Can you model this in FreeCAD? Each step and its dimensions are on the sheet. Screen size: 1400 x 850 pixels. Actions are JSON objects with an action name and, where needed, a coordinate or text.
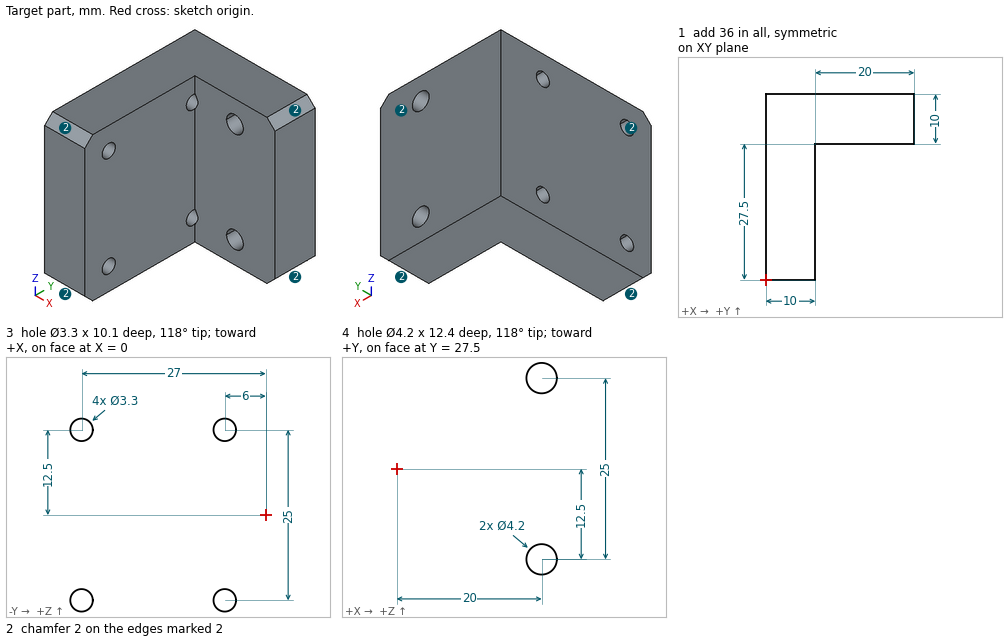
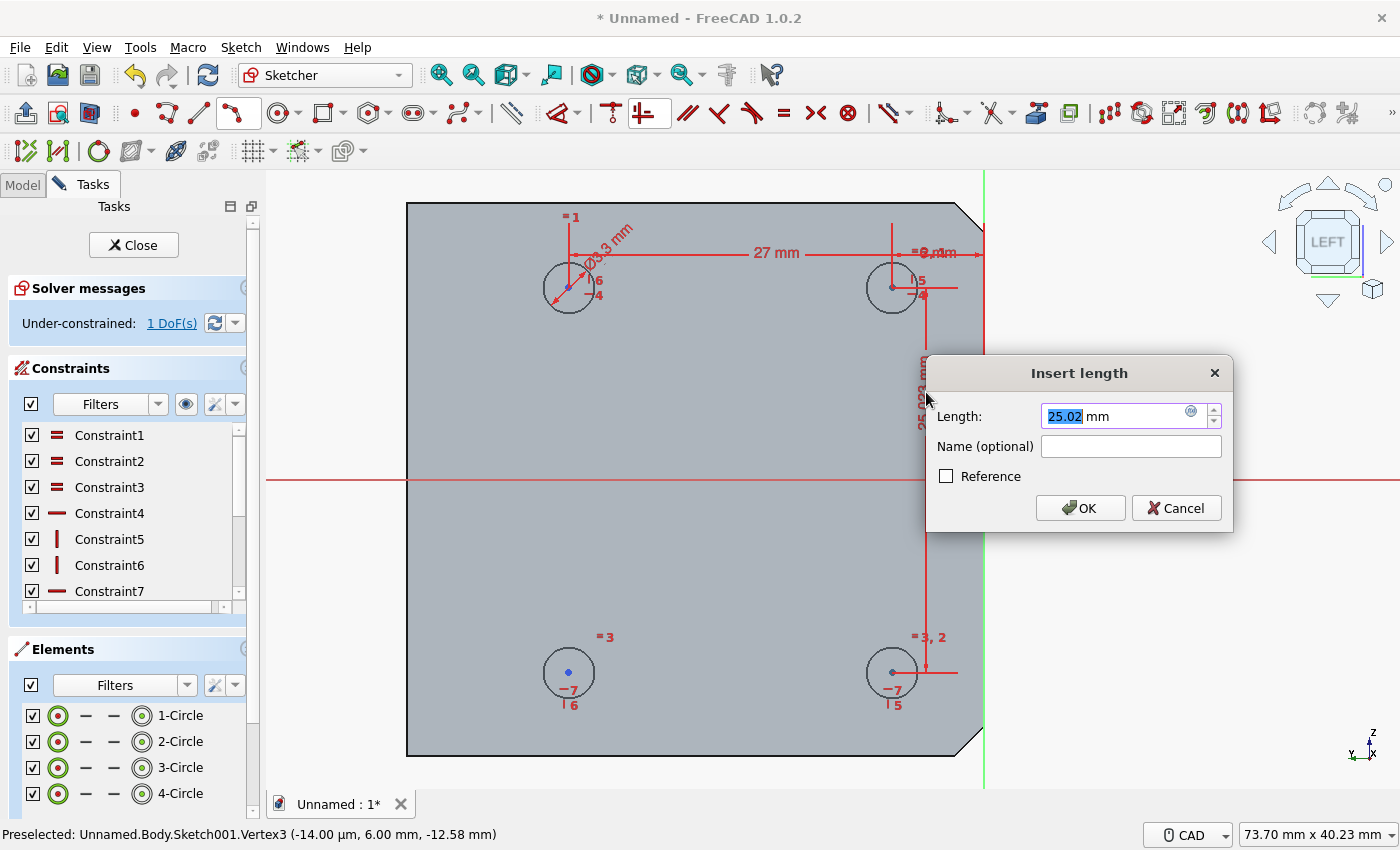
{"action": "type", "text": "25"}
{"action": "key", "text": "Return"}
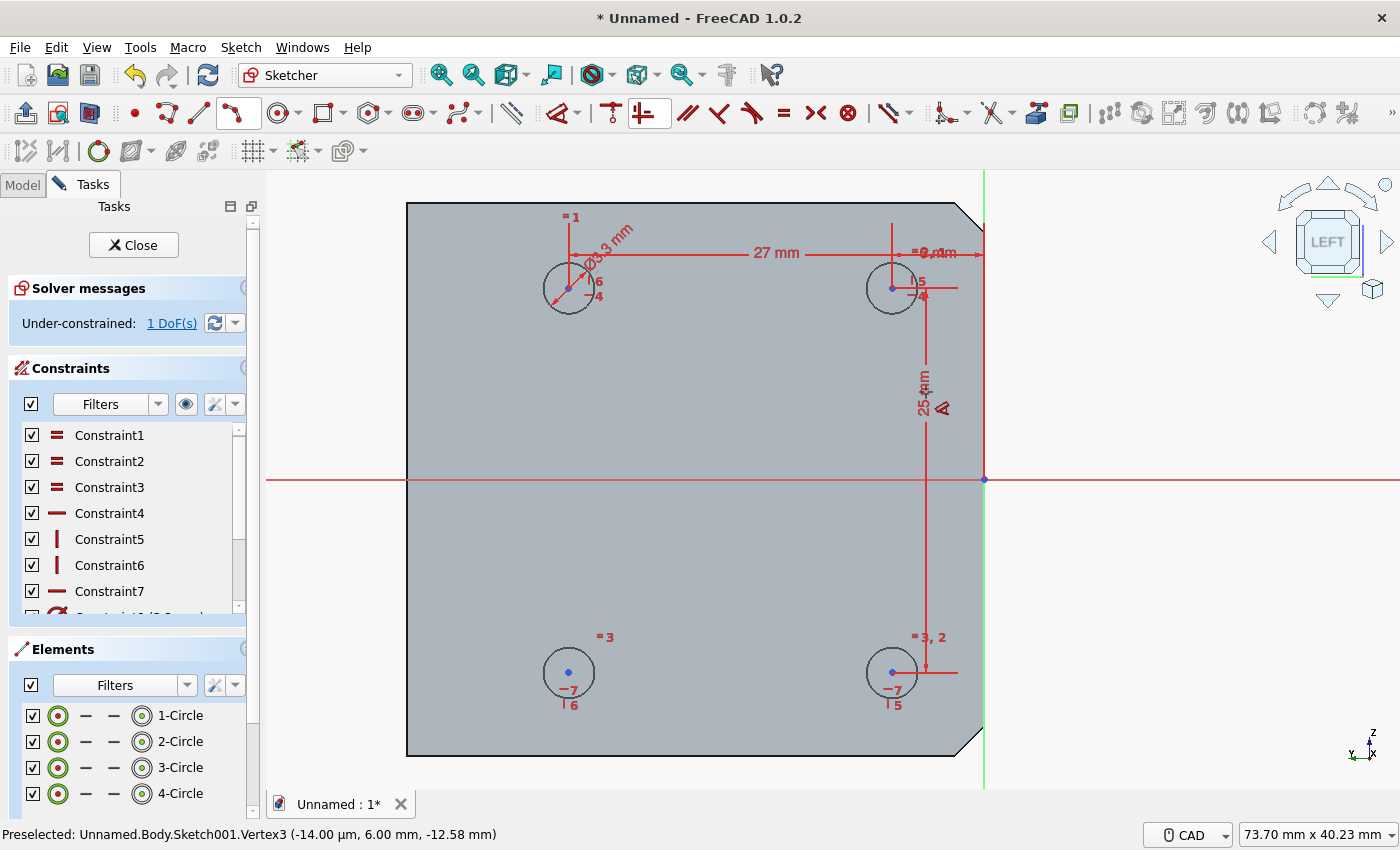
{"action": "left_click", "coordinate": [569, 288]}
{"action": "left_click", "coordinate": [1018, 384]}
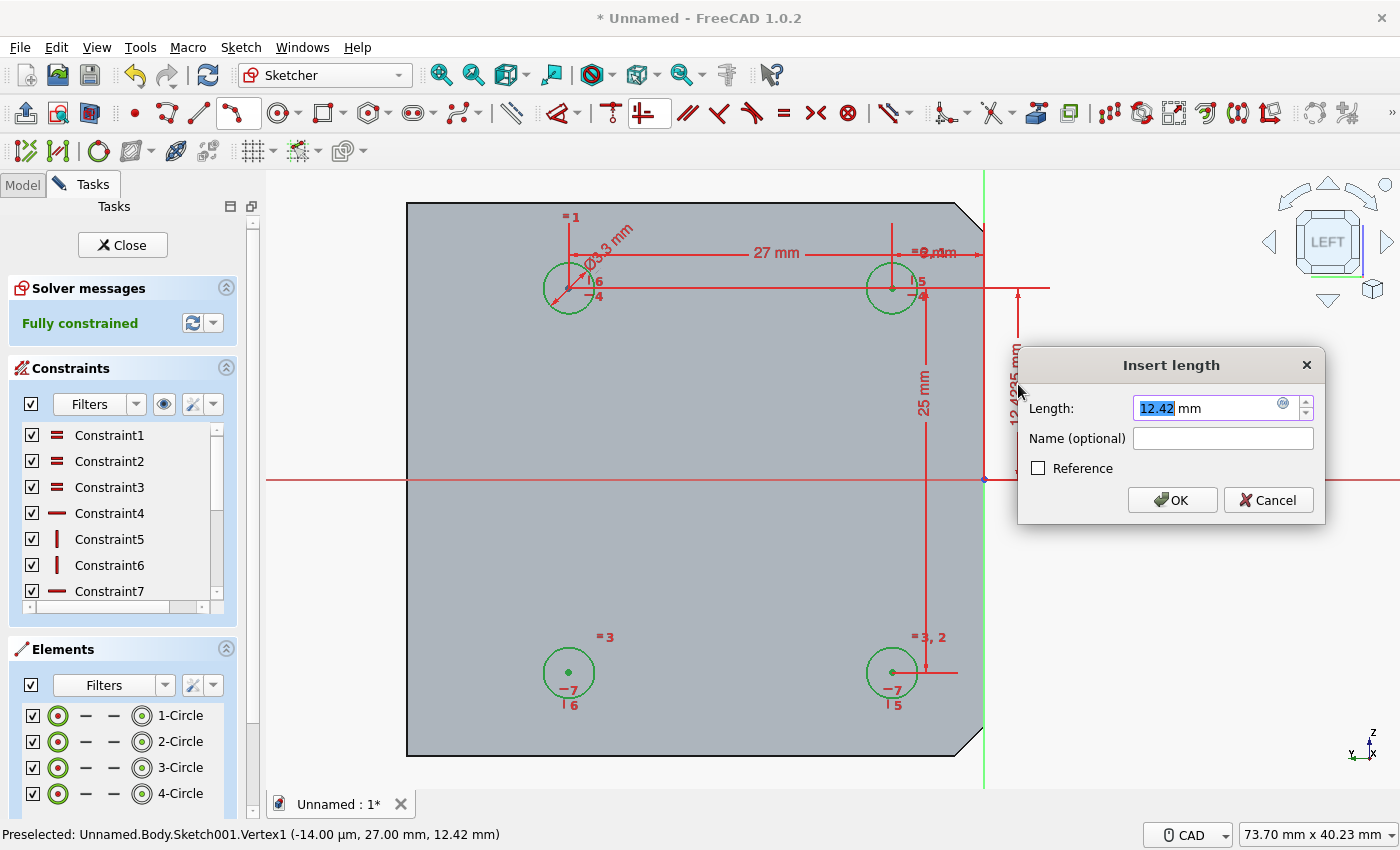
{"action": "type", "text": "12.5"}
{"action": "key", "text": "Return"}
{"action": "key", "text": "Escape"}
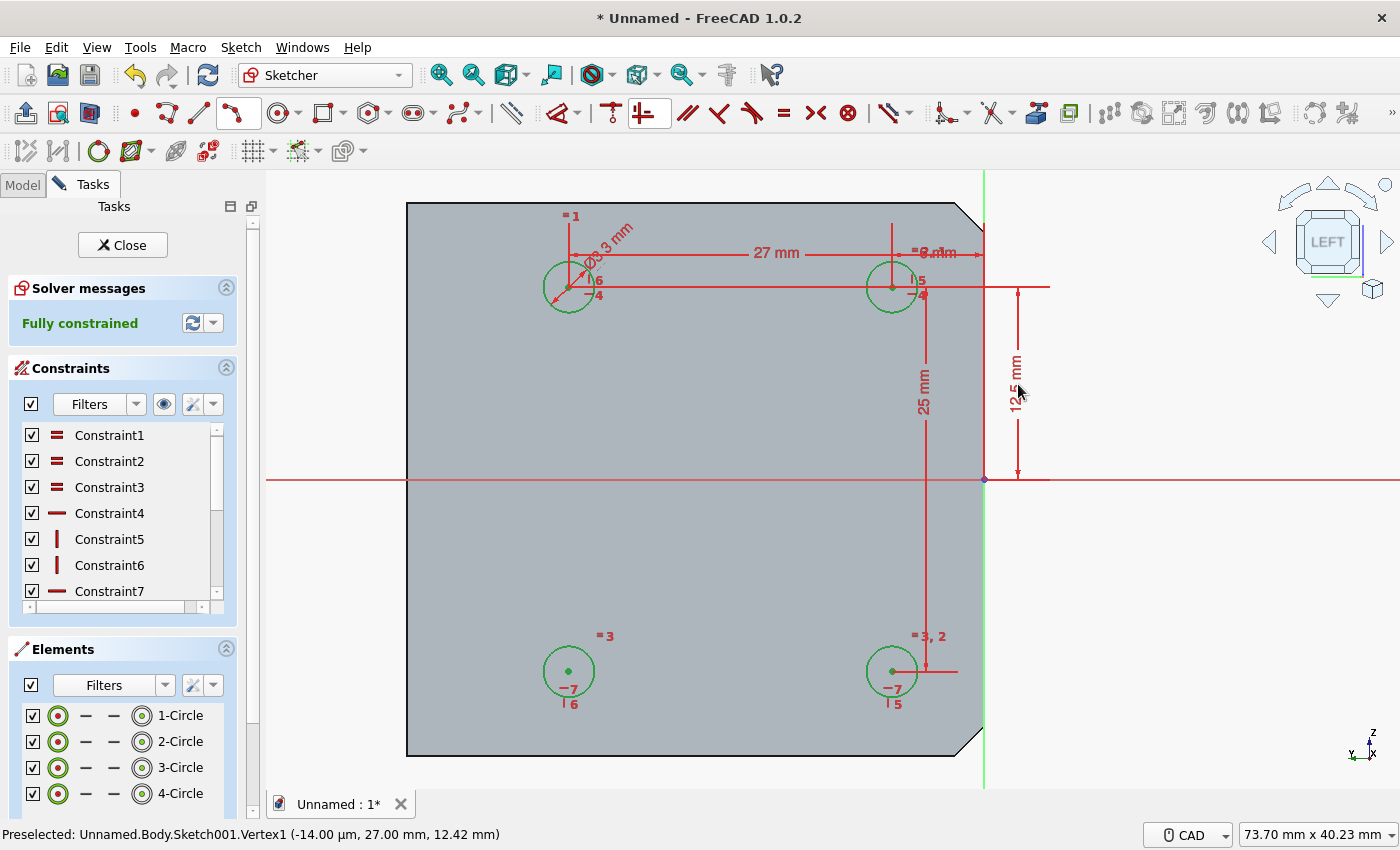
{"action": "left_click", "coordinate": [123, 245]}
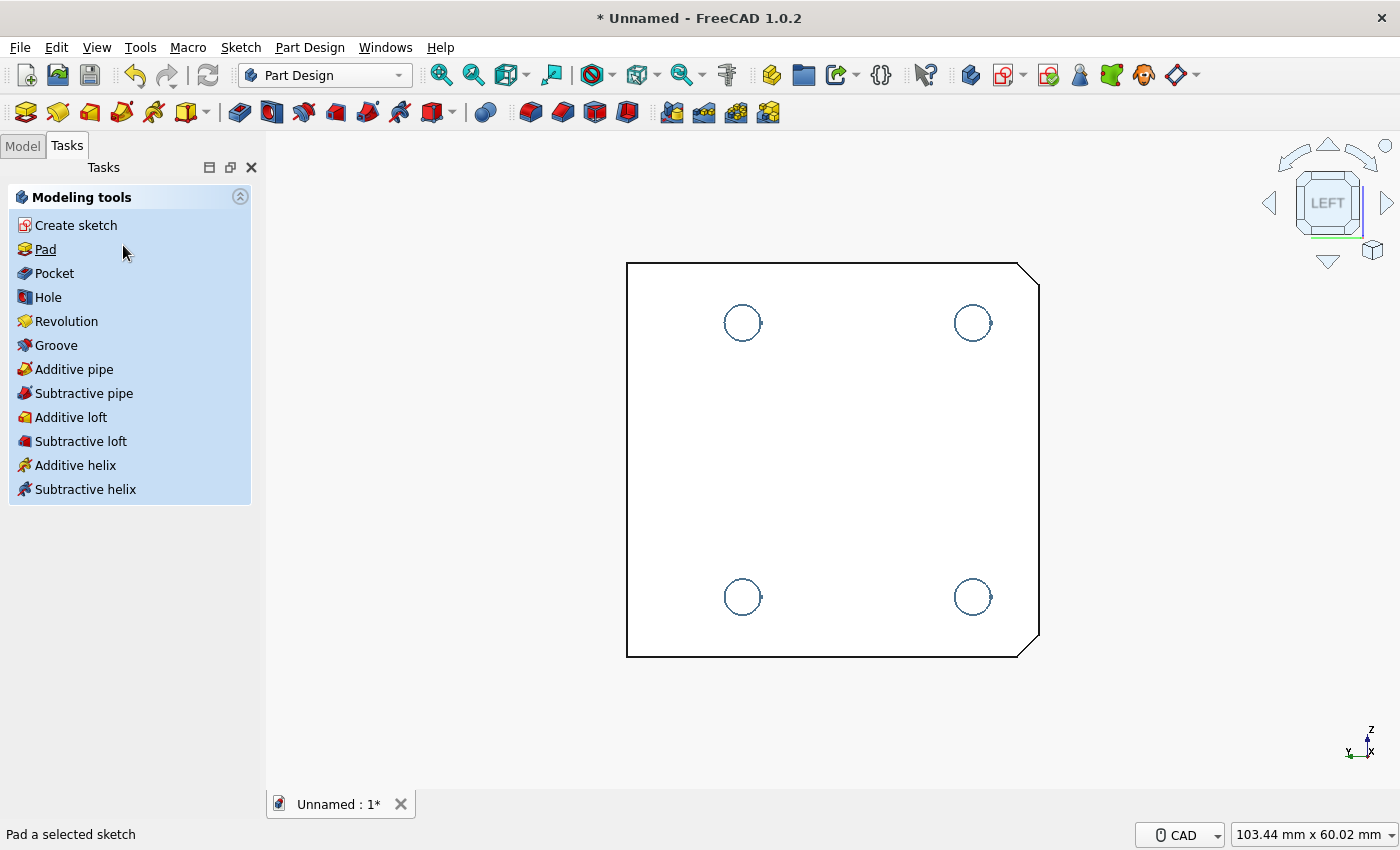
{"action": "left_click", "coordinate": [272, 112]}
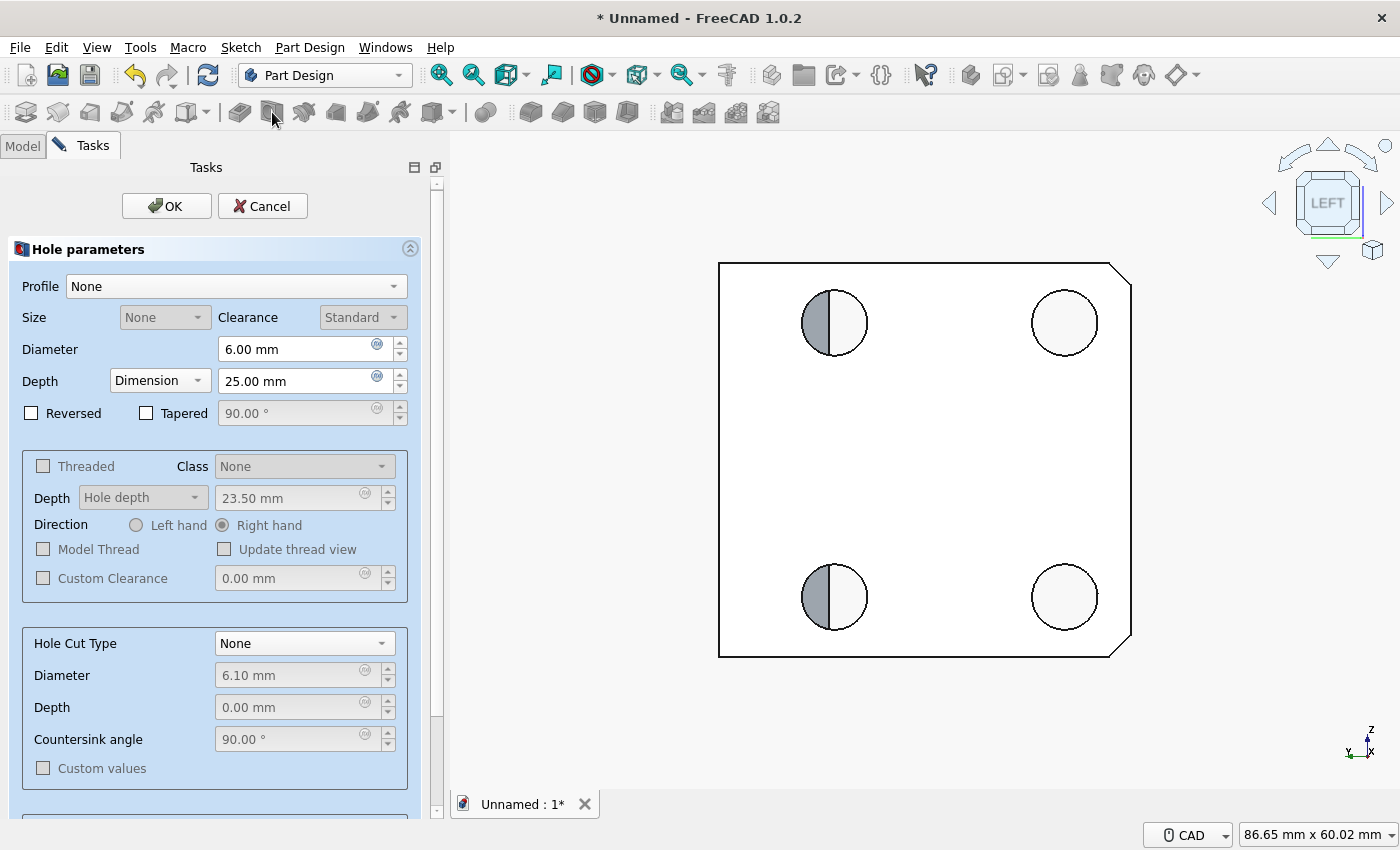
{"action": "triple_click", "coordinate": [305, 349]}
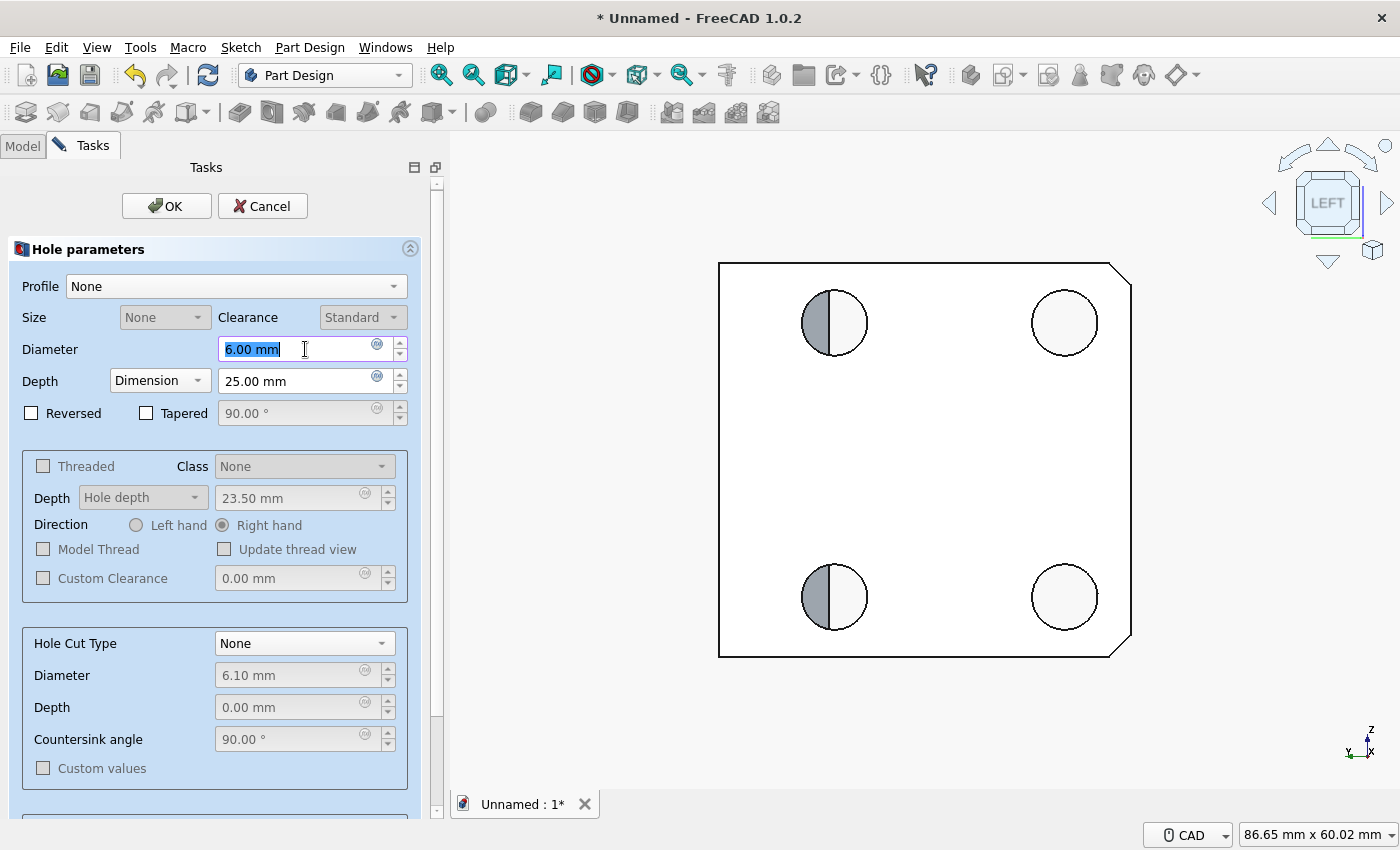
{"action": "type", "text": "3.3"}
{"action": "key", "text": "Tab"}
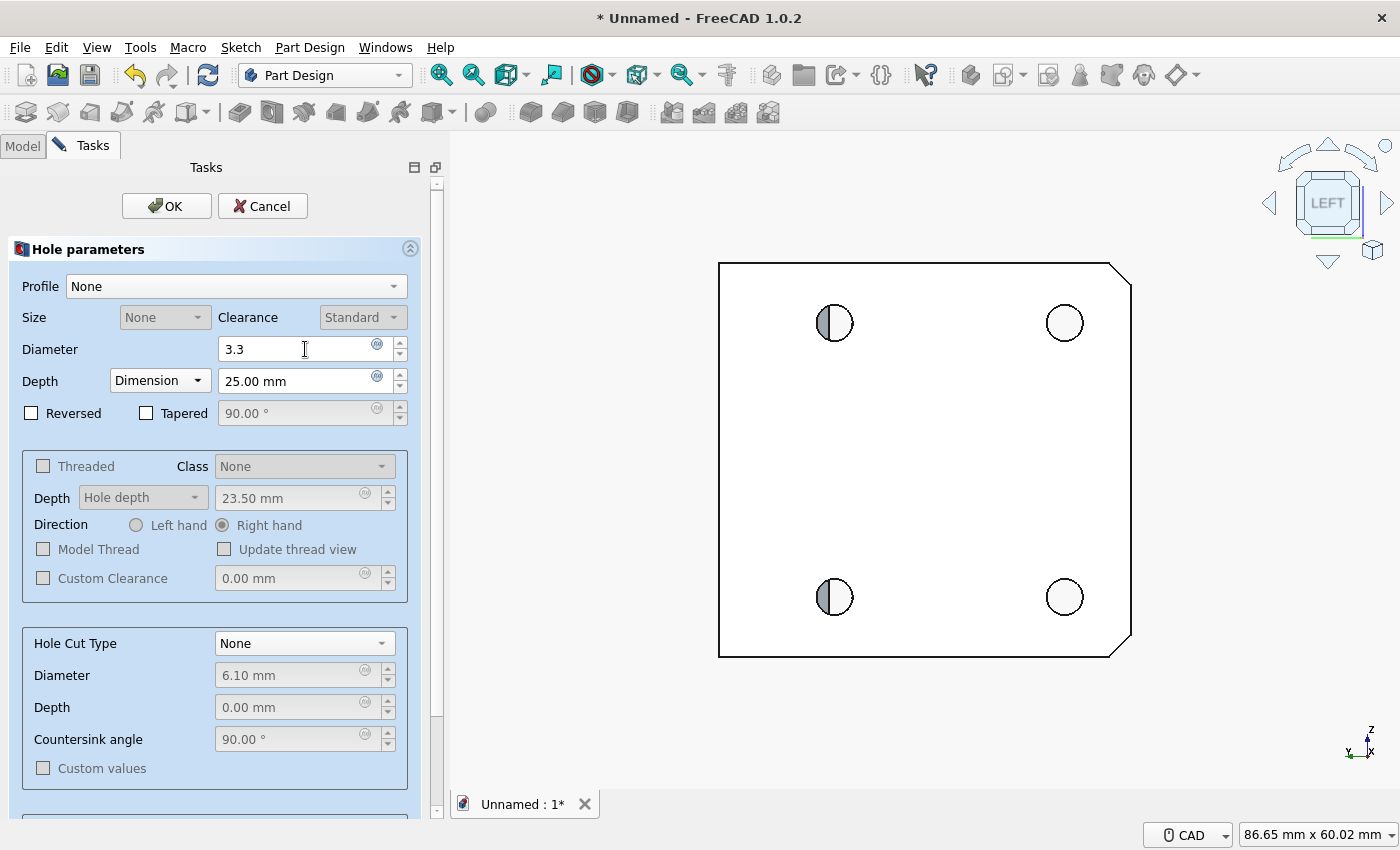
{"action": "triple_click", "coordinate": [305, 381]}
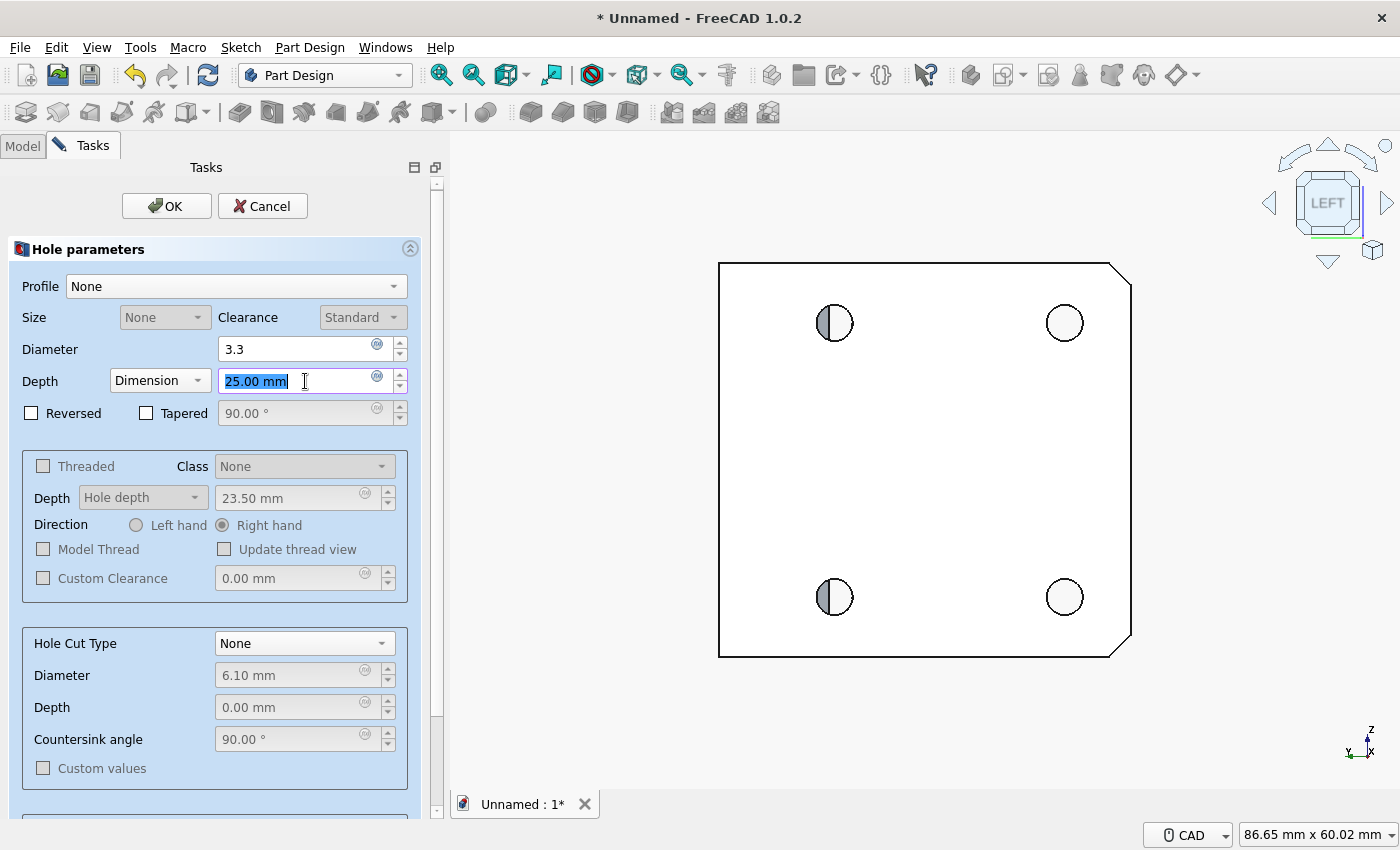
{"action": "type", "text": "10.1"}
{"action": "key", "text": "Tab"}